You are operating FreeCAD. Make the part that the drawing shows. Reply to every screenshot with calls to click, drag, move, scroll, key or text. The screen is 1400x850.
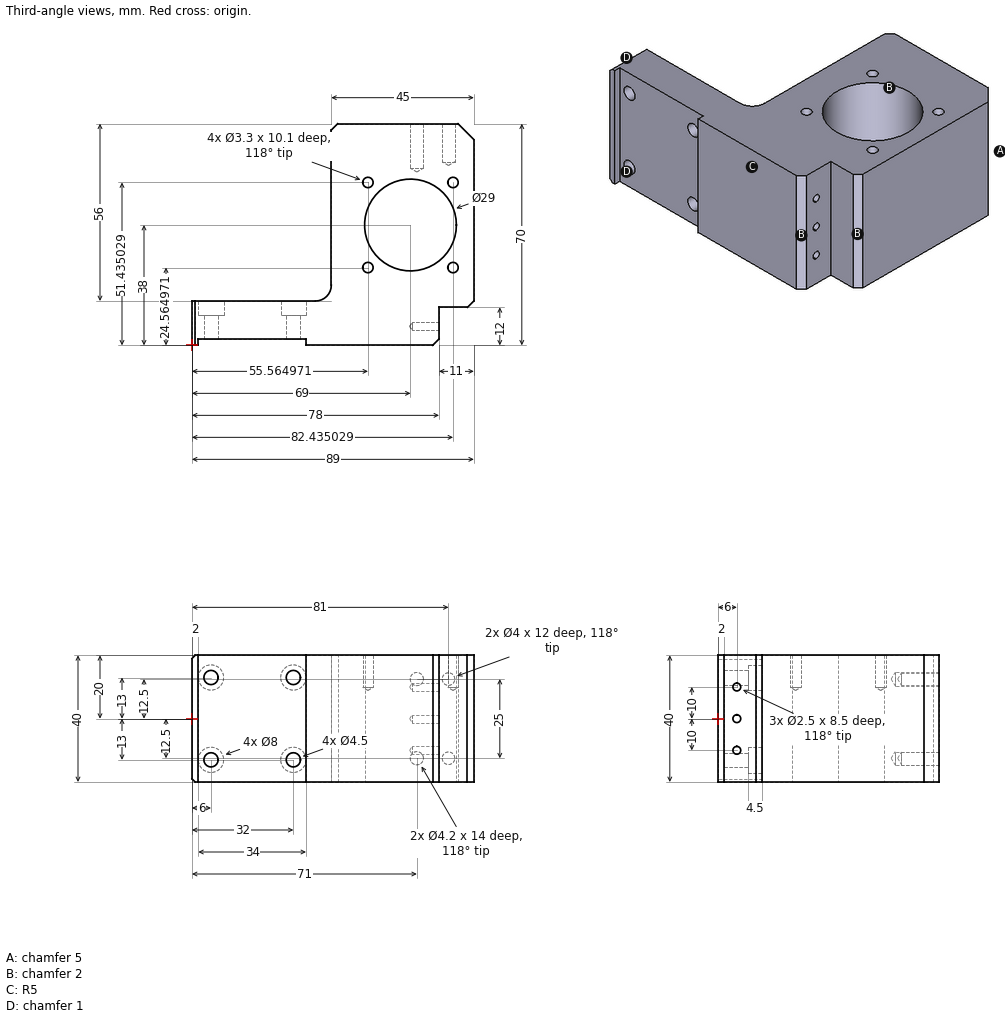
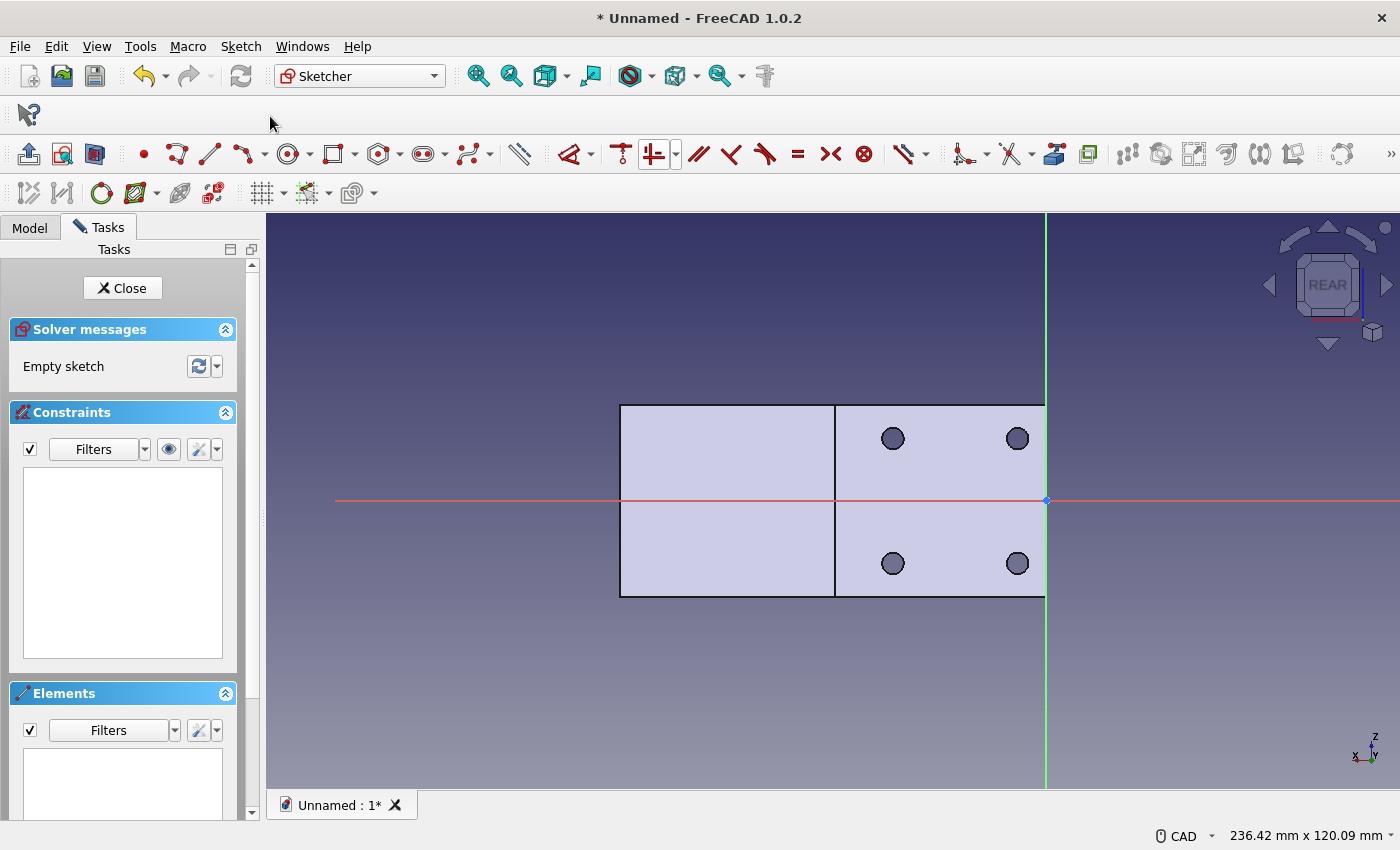
scroll(672, 501, up, 5)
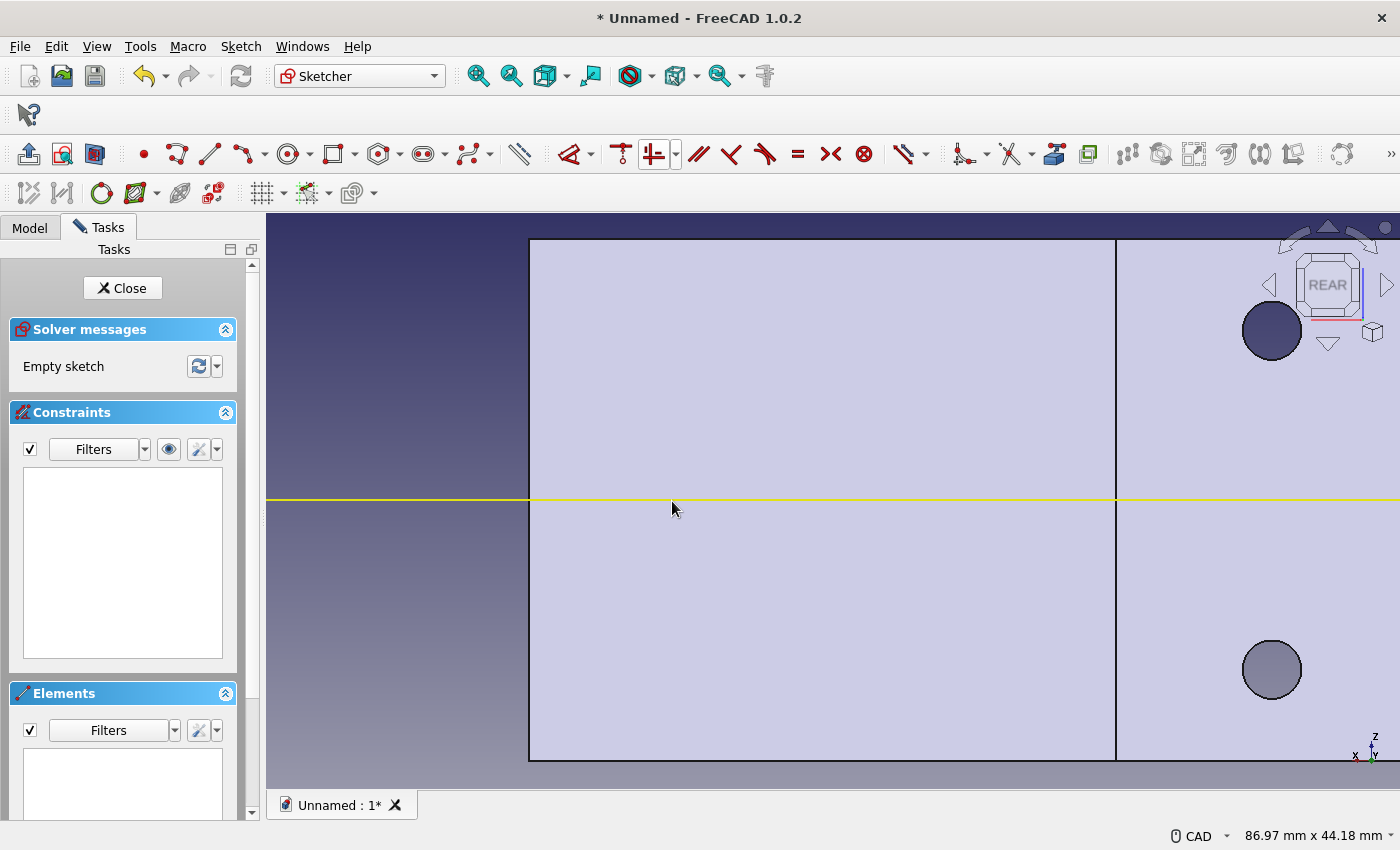
click(288, 154)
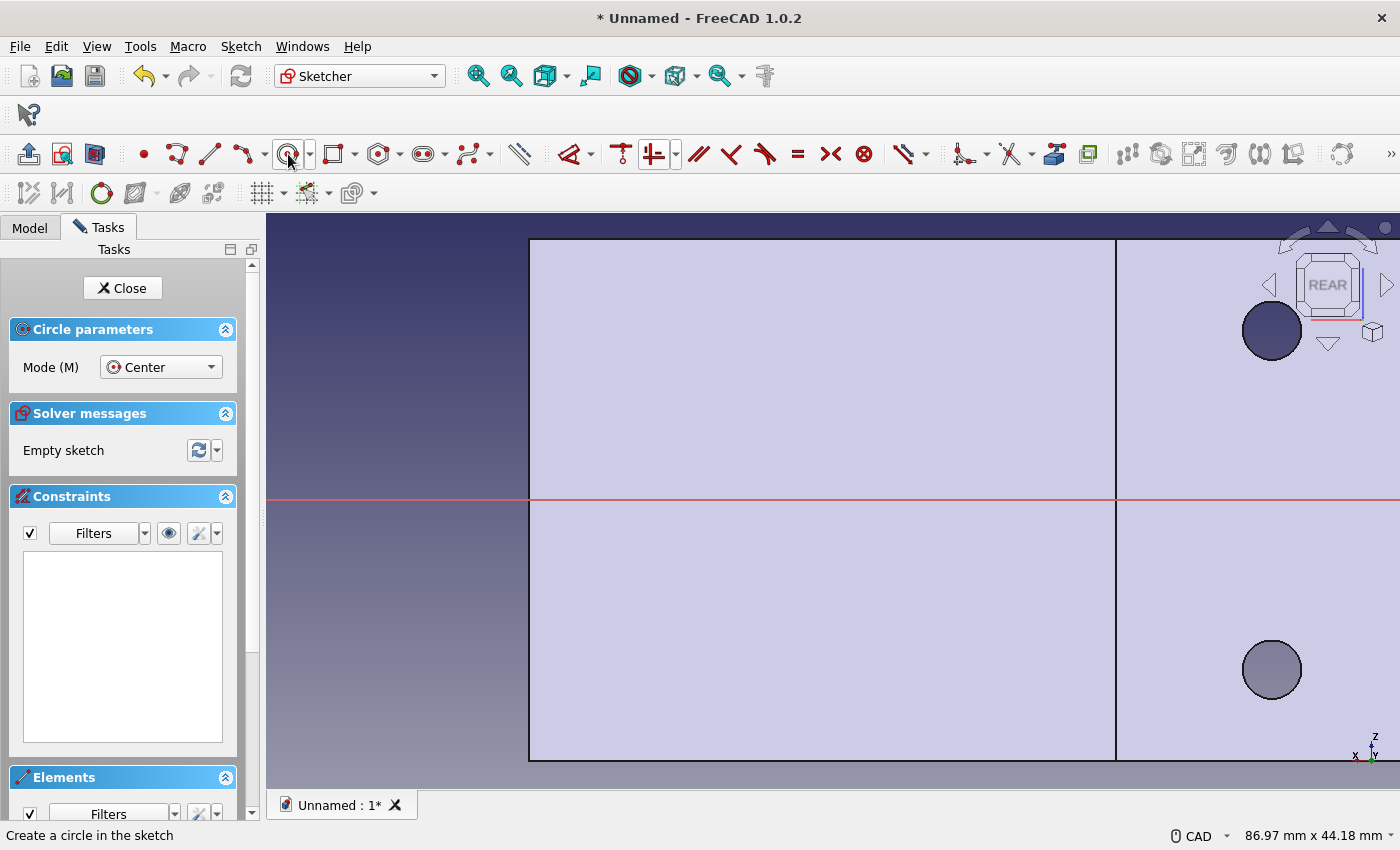
click(764, 663)
move(783, 644)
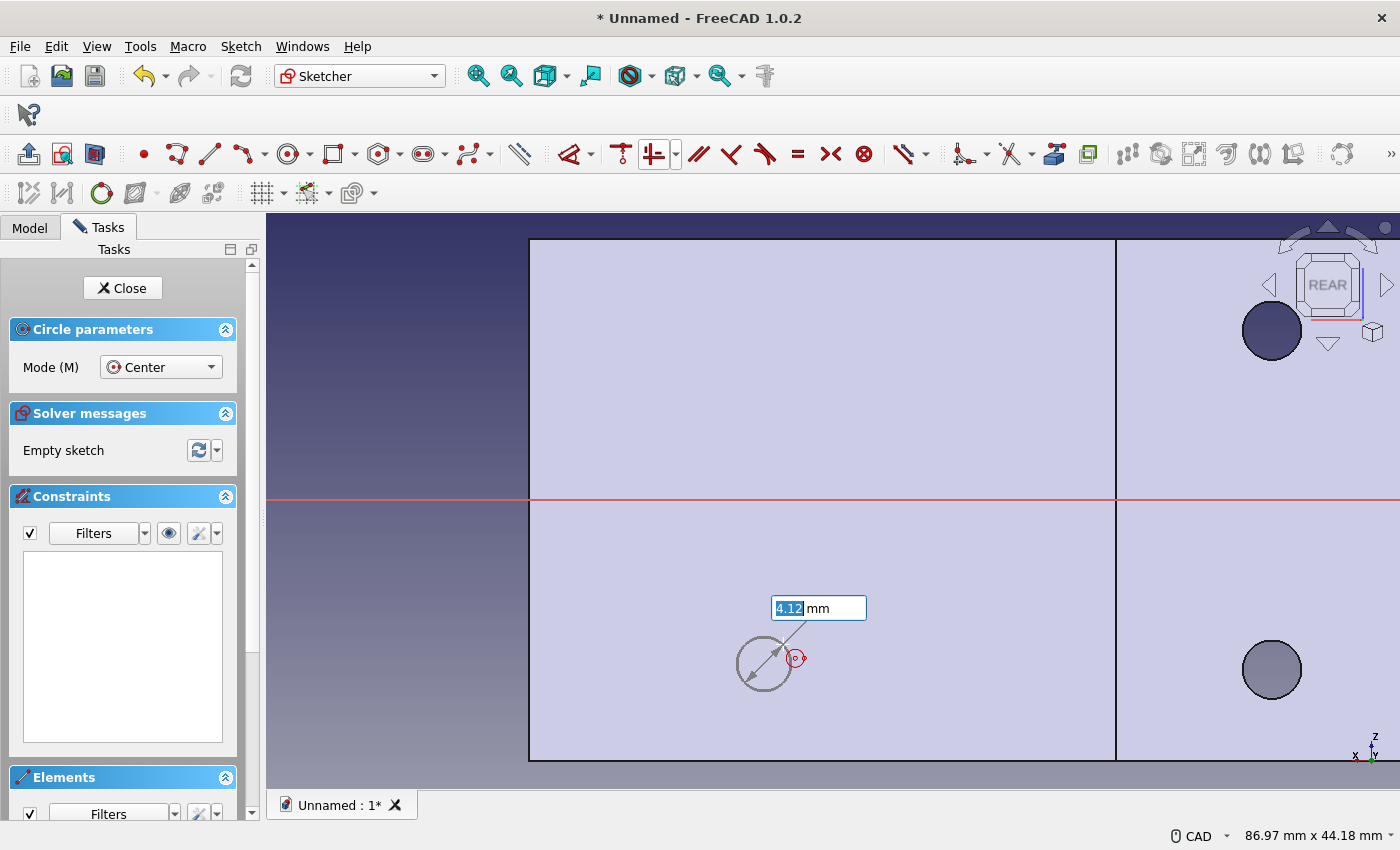
text(4.2)
key(Return)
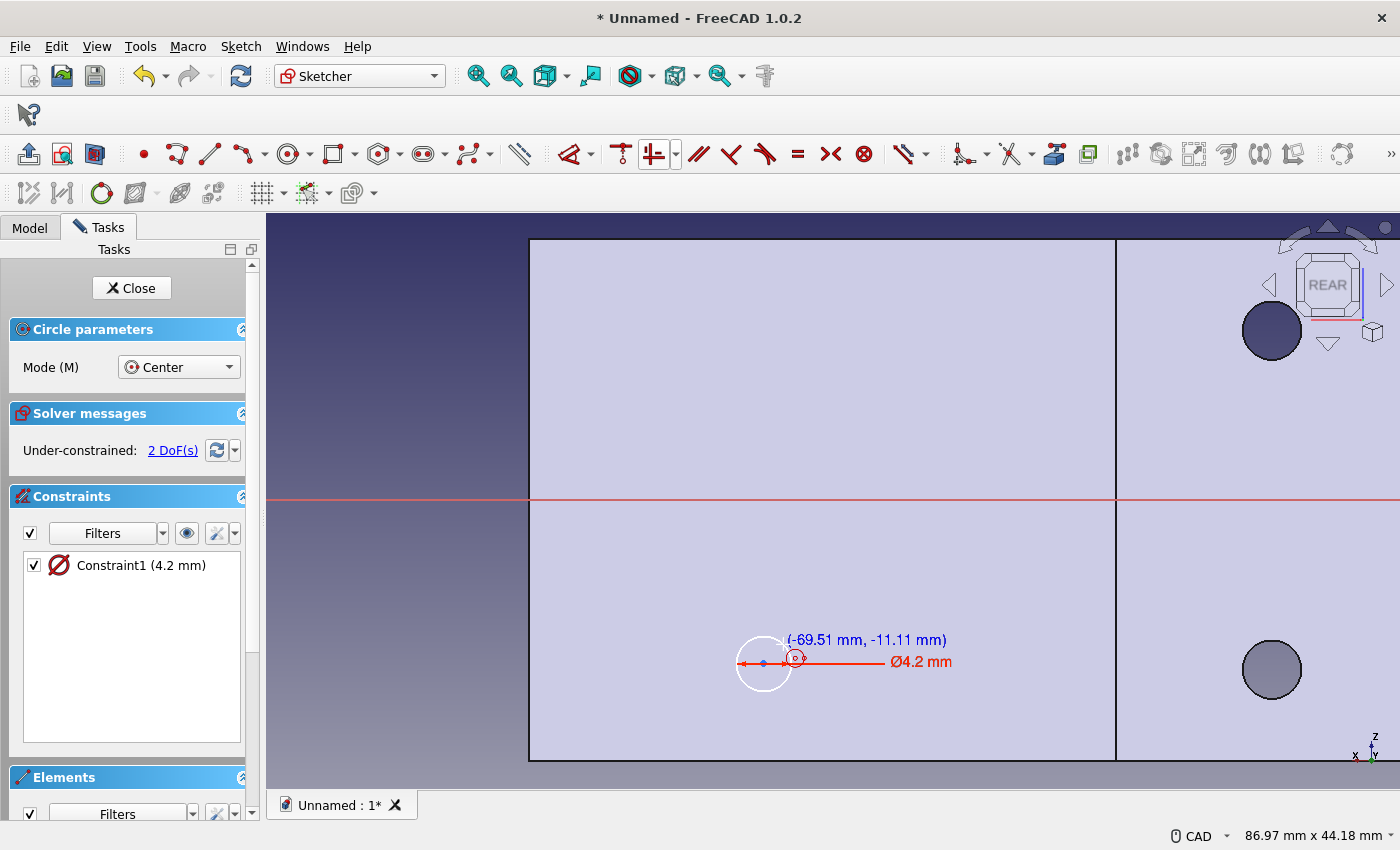
click(764, 337)
move(783, 318)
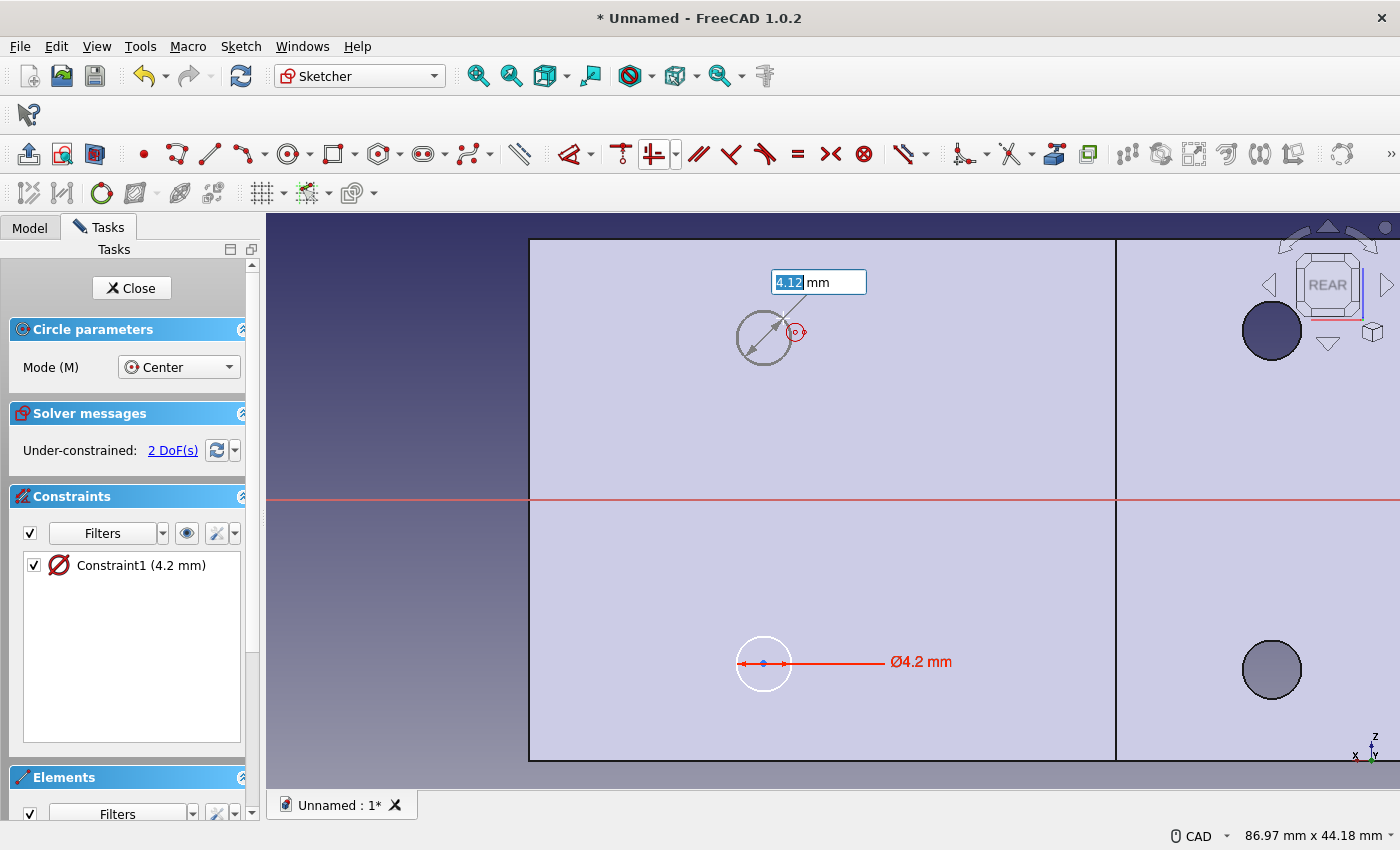
text(4.2)
key(Return)
key(Escape)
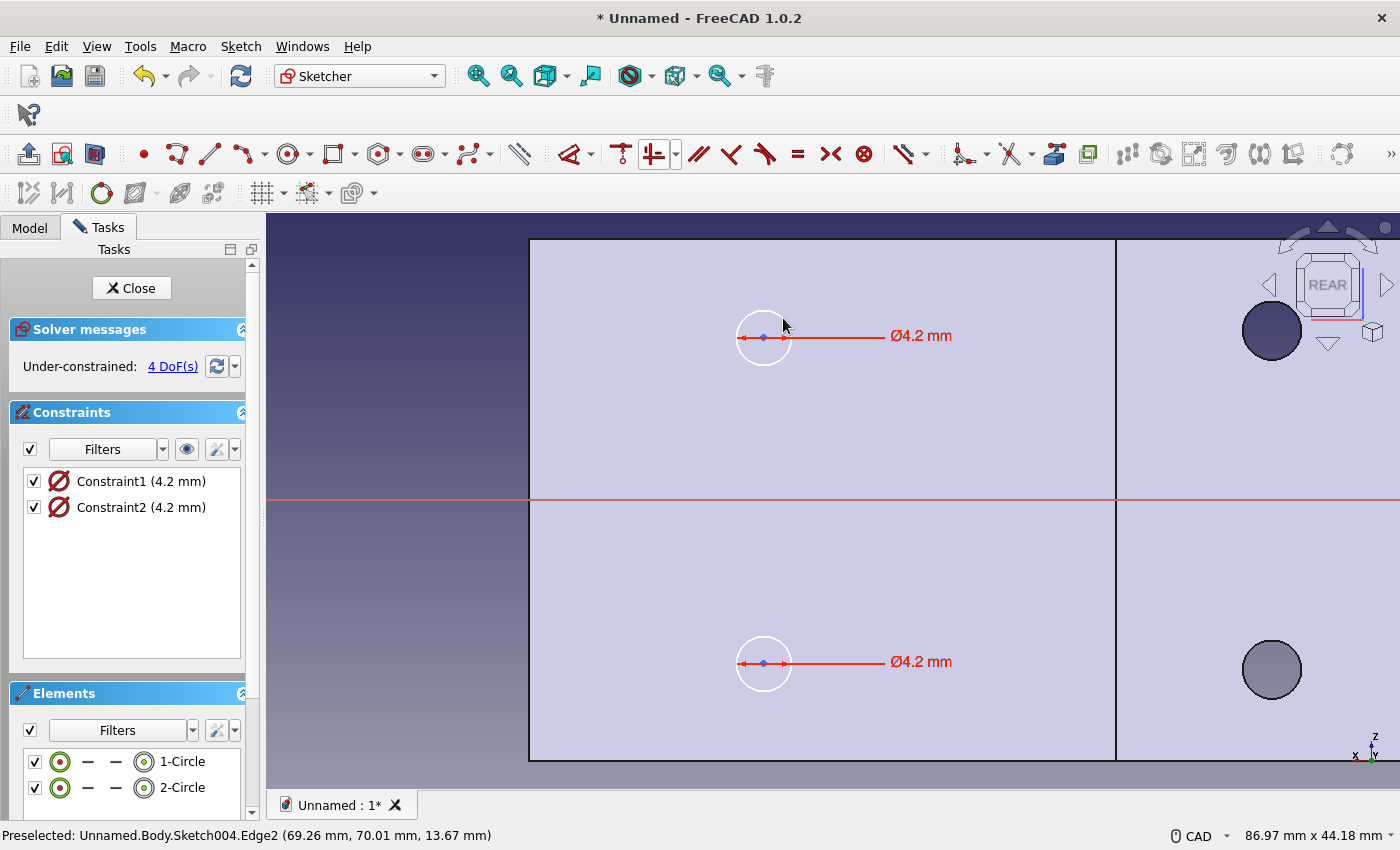
click(764, 664)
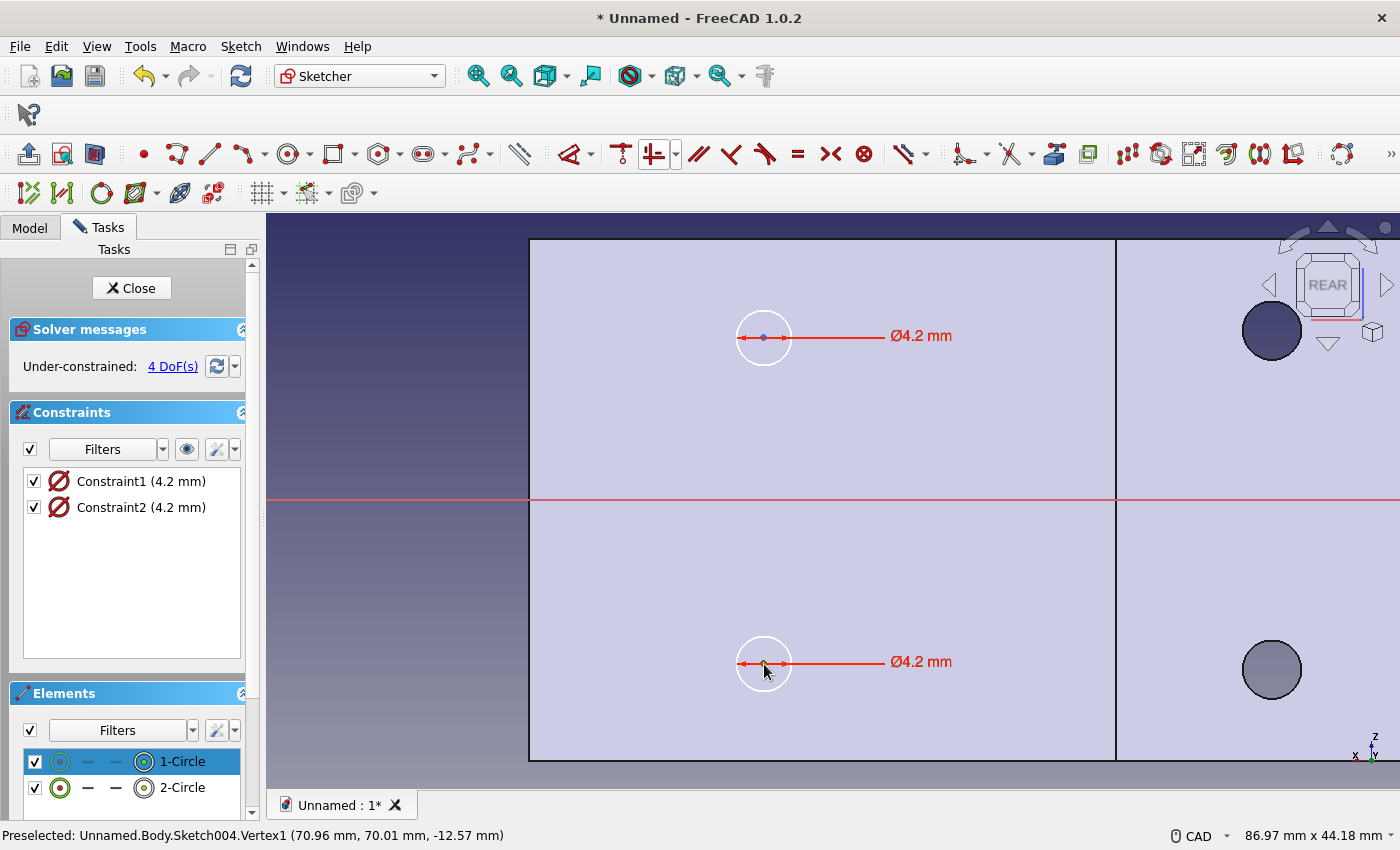
click(764, 338)